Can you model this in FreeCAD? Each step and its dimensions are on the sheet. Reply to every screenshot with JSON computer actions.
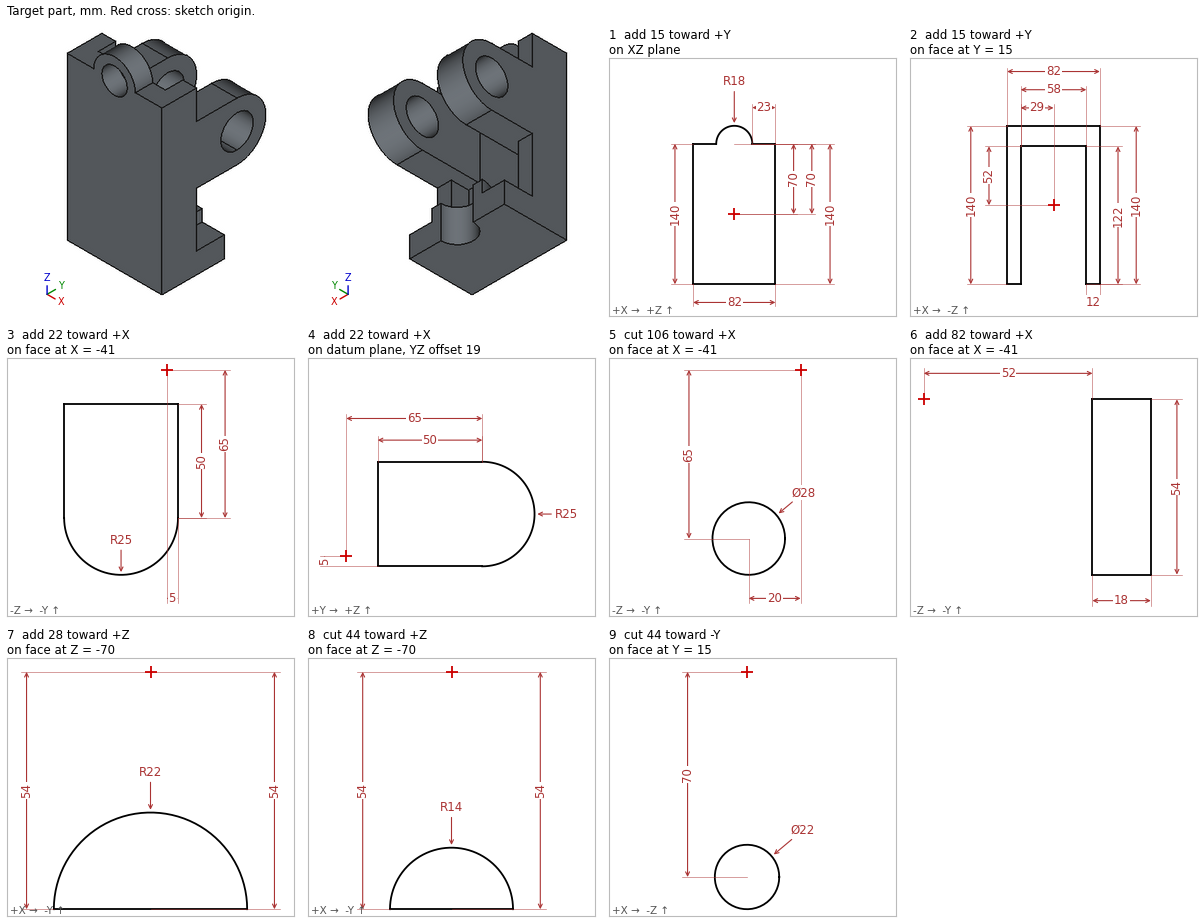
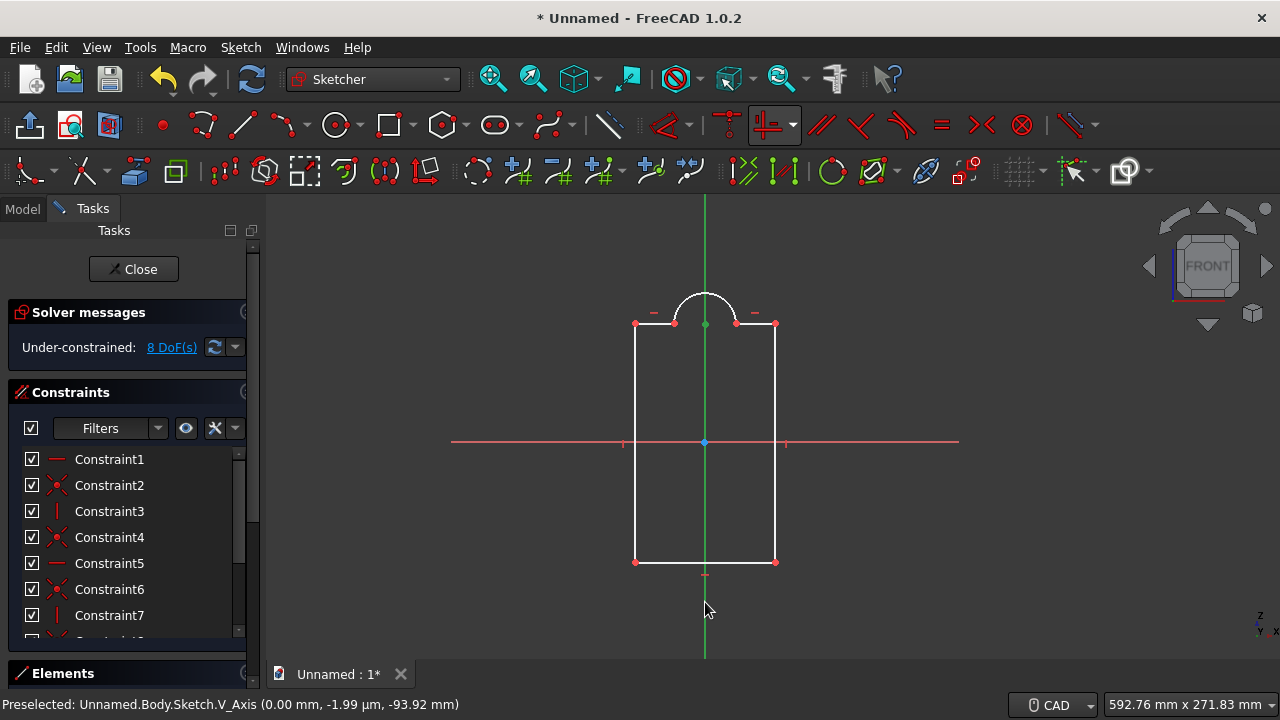
{"action": "left_click", "coordinate": [728, 126]}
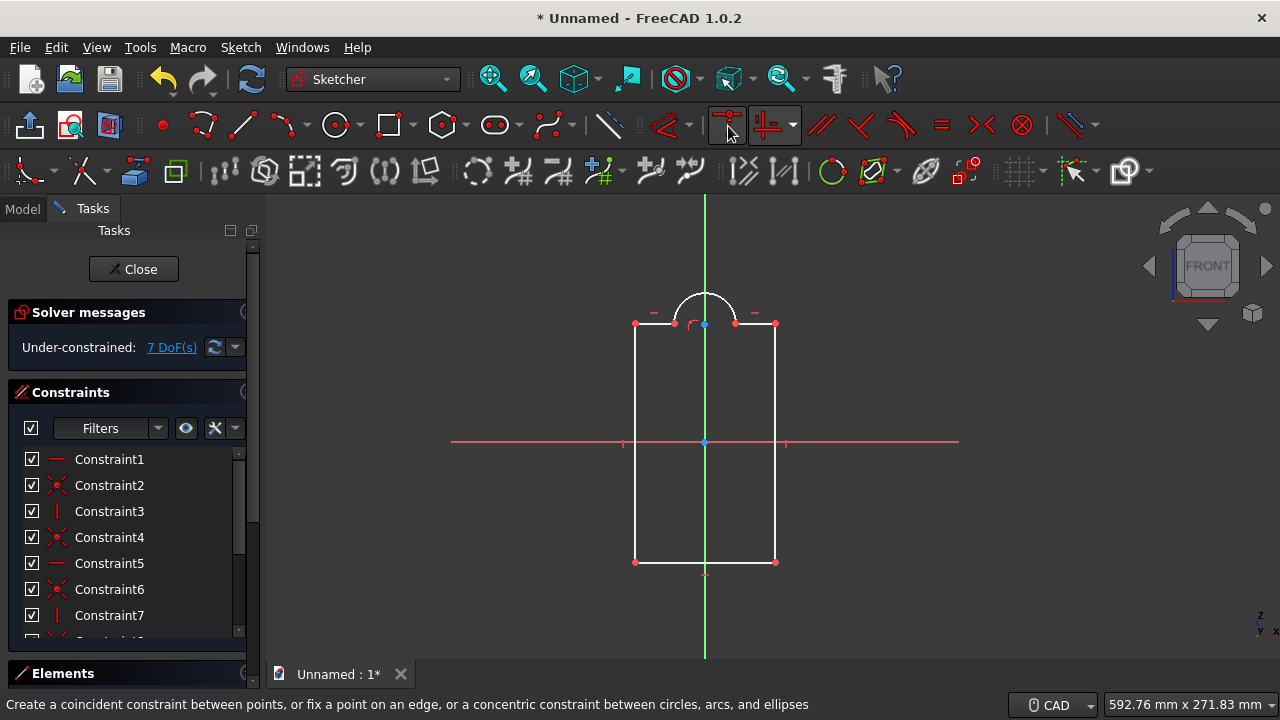
{"action": "scroll", "coordinate": [723, 299], "scroll_direction": "up", "scroll_amount": 2}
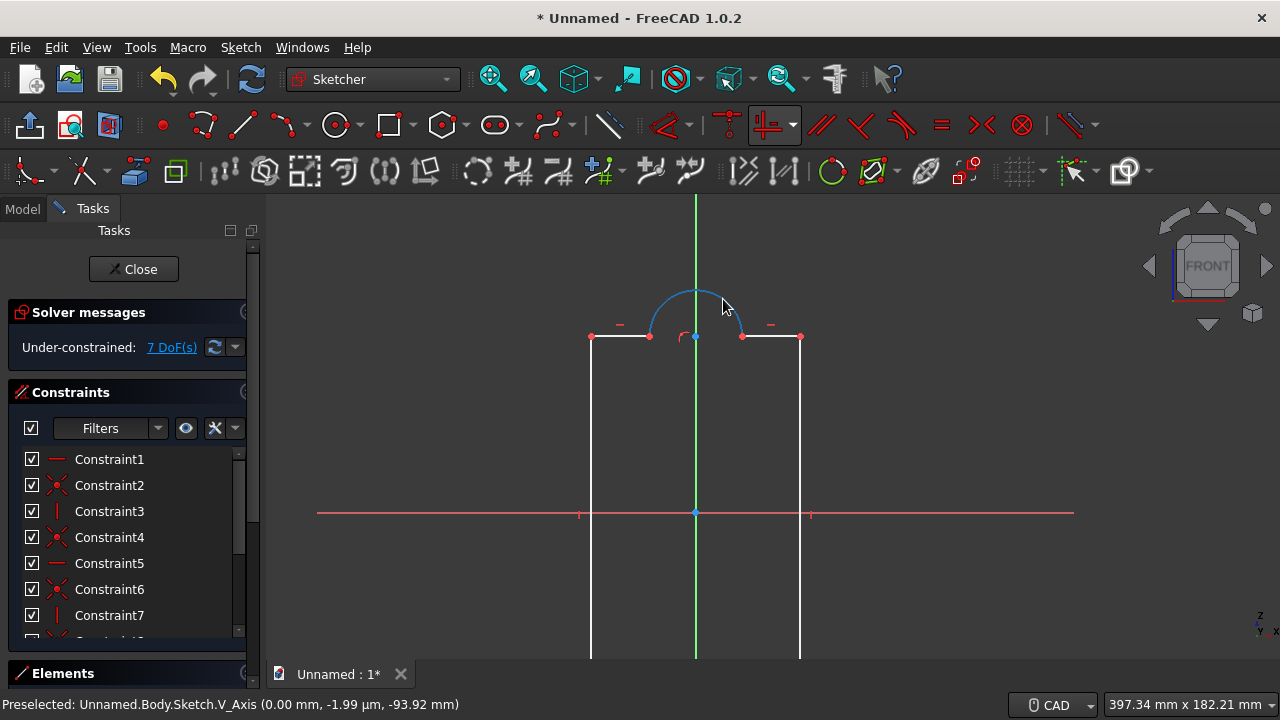
{"action": "left_click", "coordinate": [723, 299]}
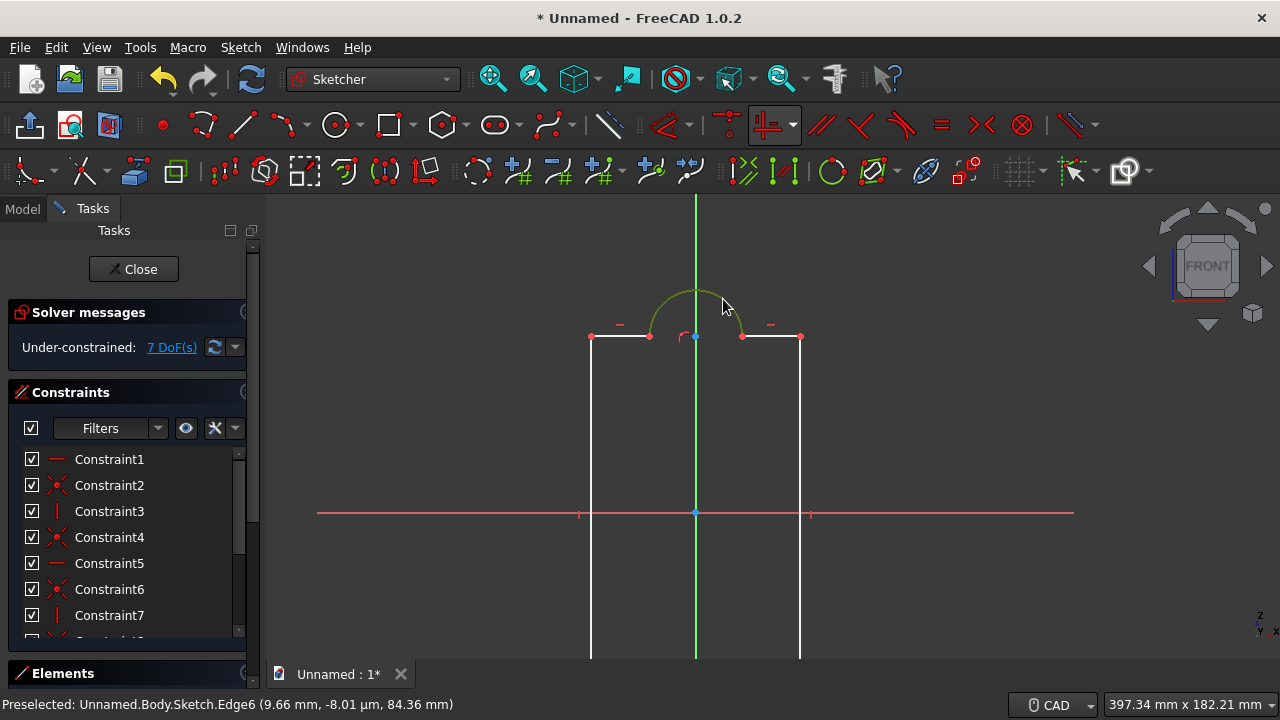
{"action": "key", "text": "k r"}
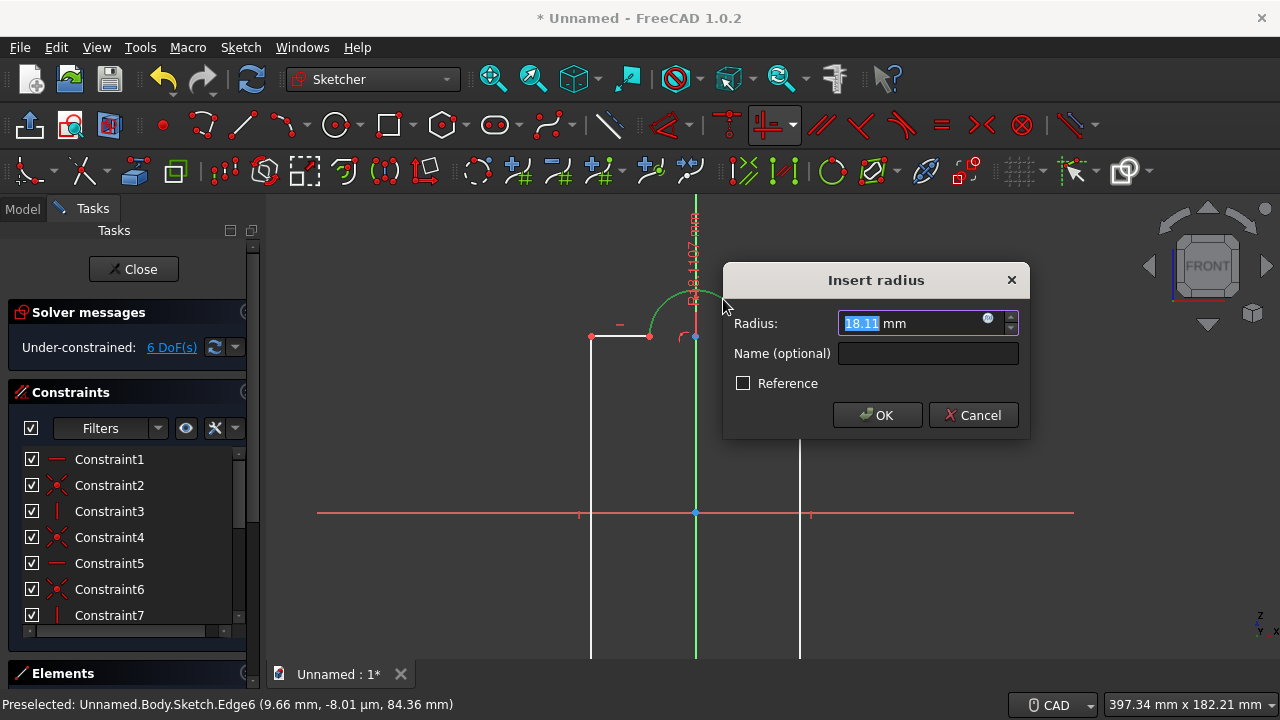
{"action": "type", "text": "18"}
{"action": "key", "text": "Return"}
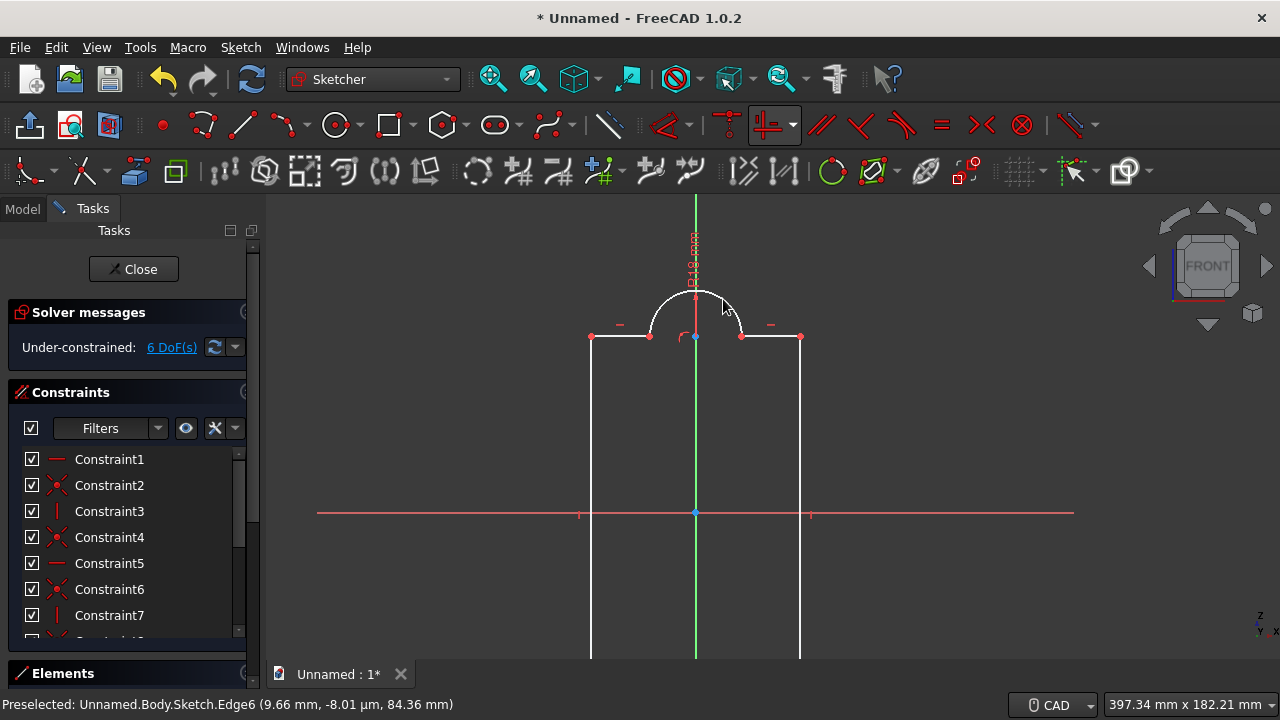
{"action": "left_click", "coordinate": [759, 336]}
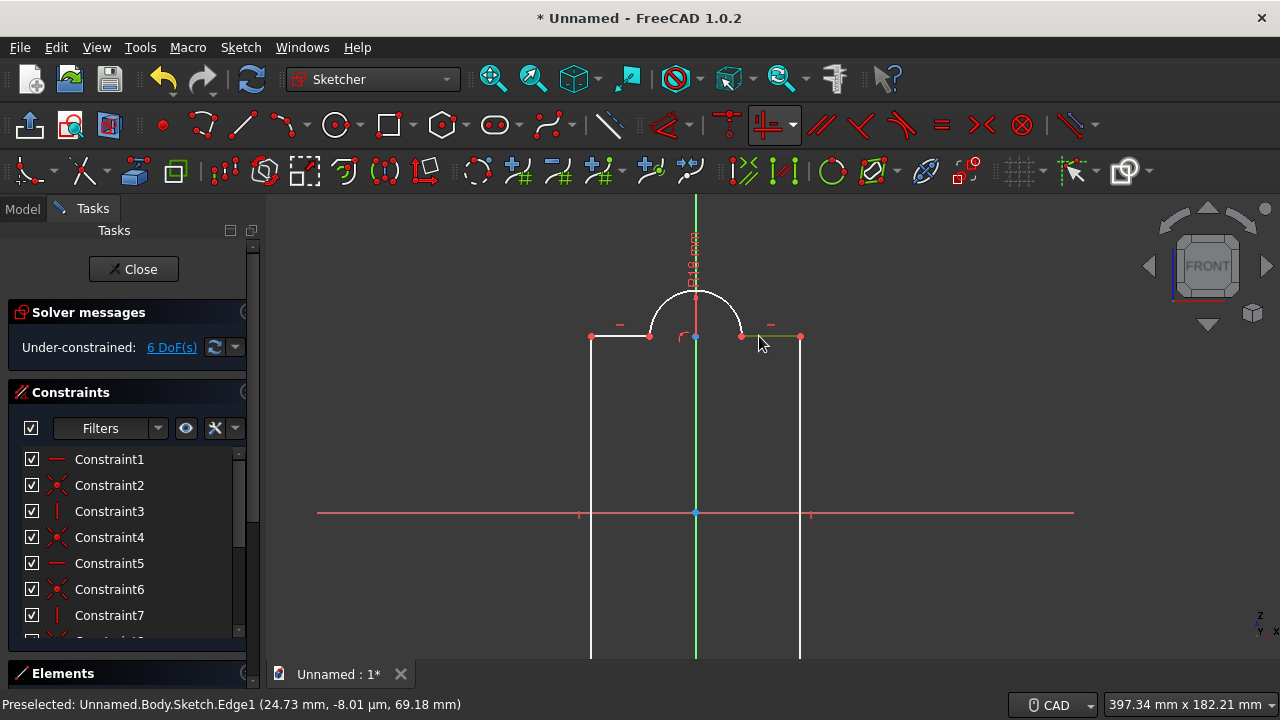
{"action": "key", "text": "l"}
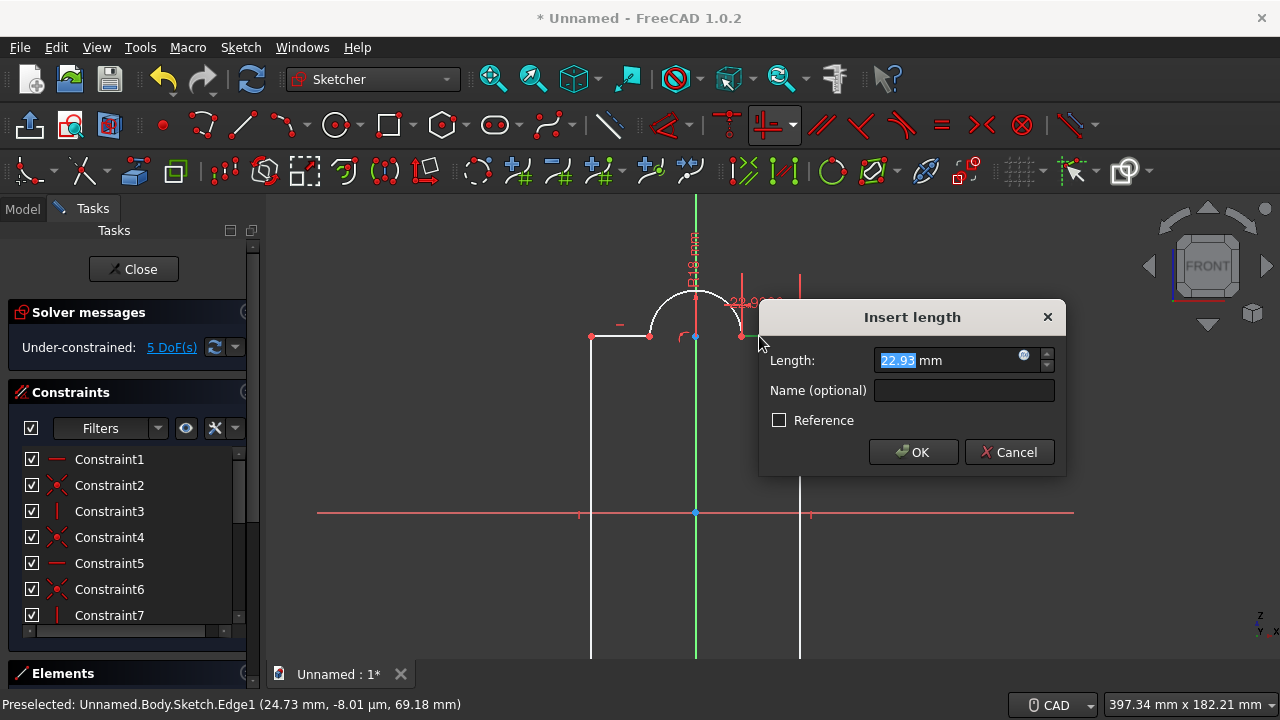
{"action": "type", "text": "23"}
{"action": "key", "text": "Return"}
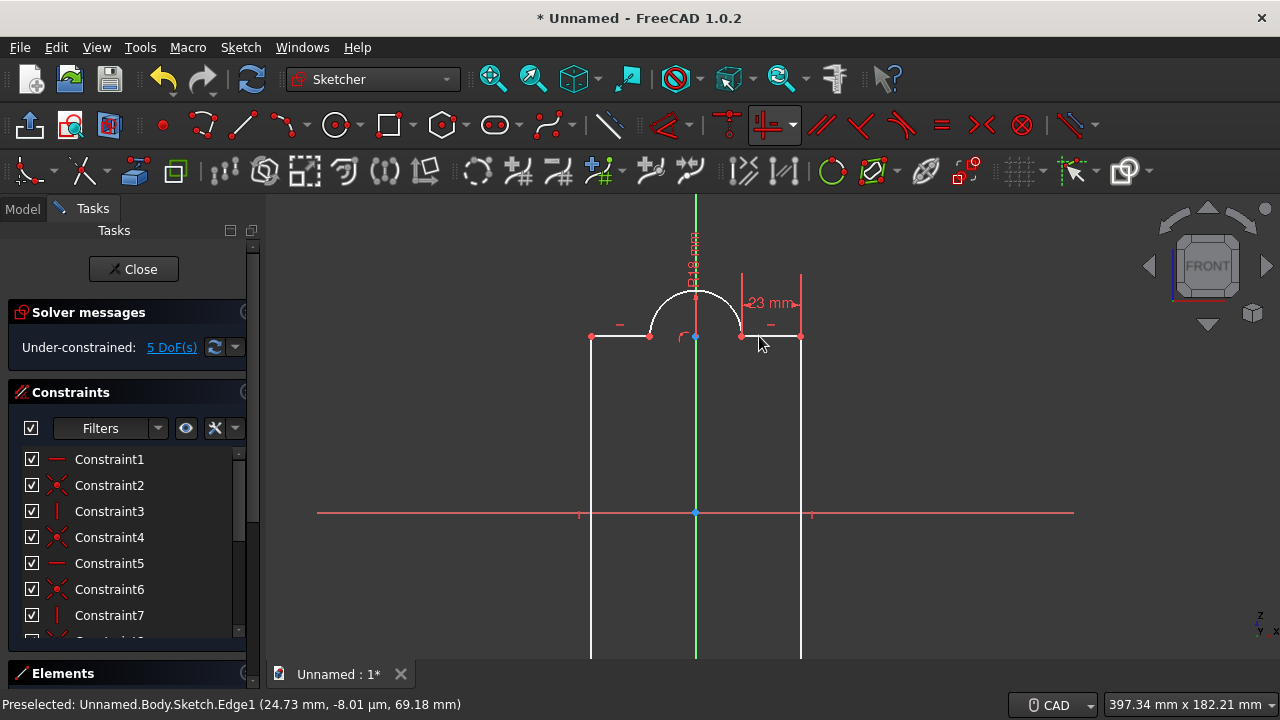
{"action": "scroll", "coordinate": [722, 298], "scroll_direction": "down", "scroll_amount": 2}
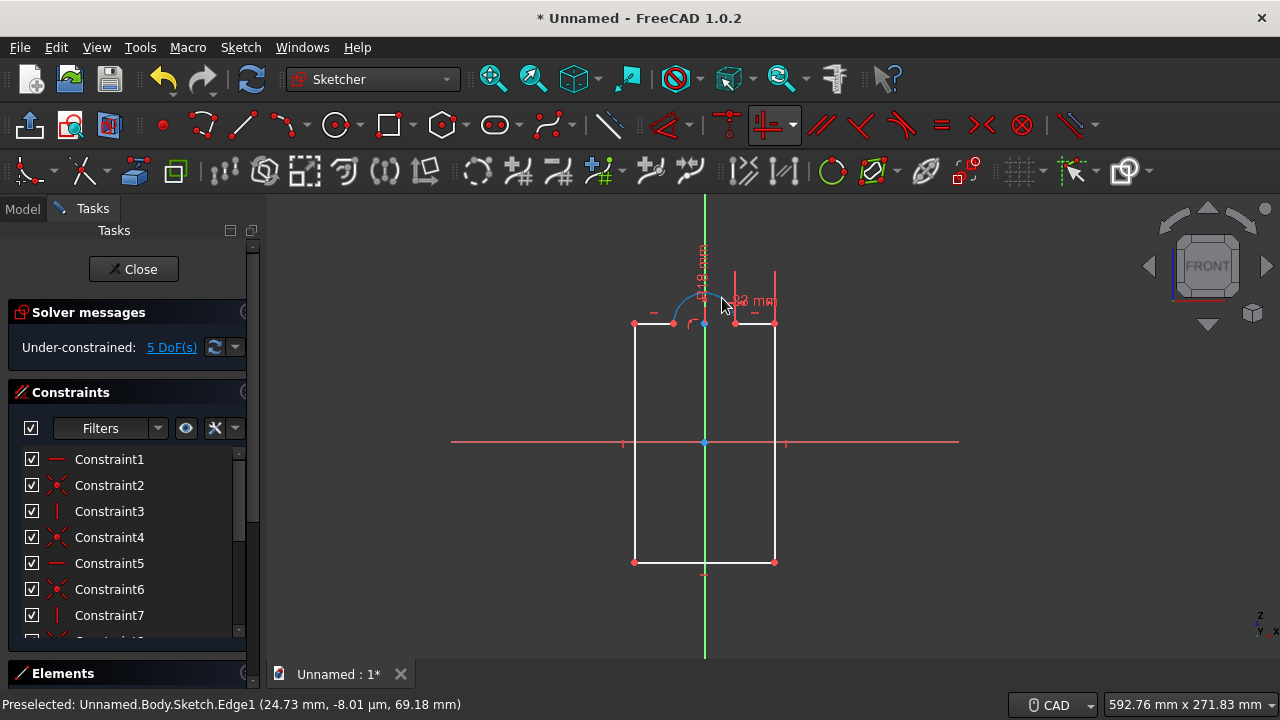
{"action": "left_click", "coordinate": [733, 563]}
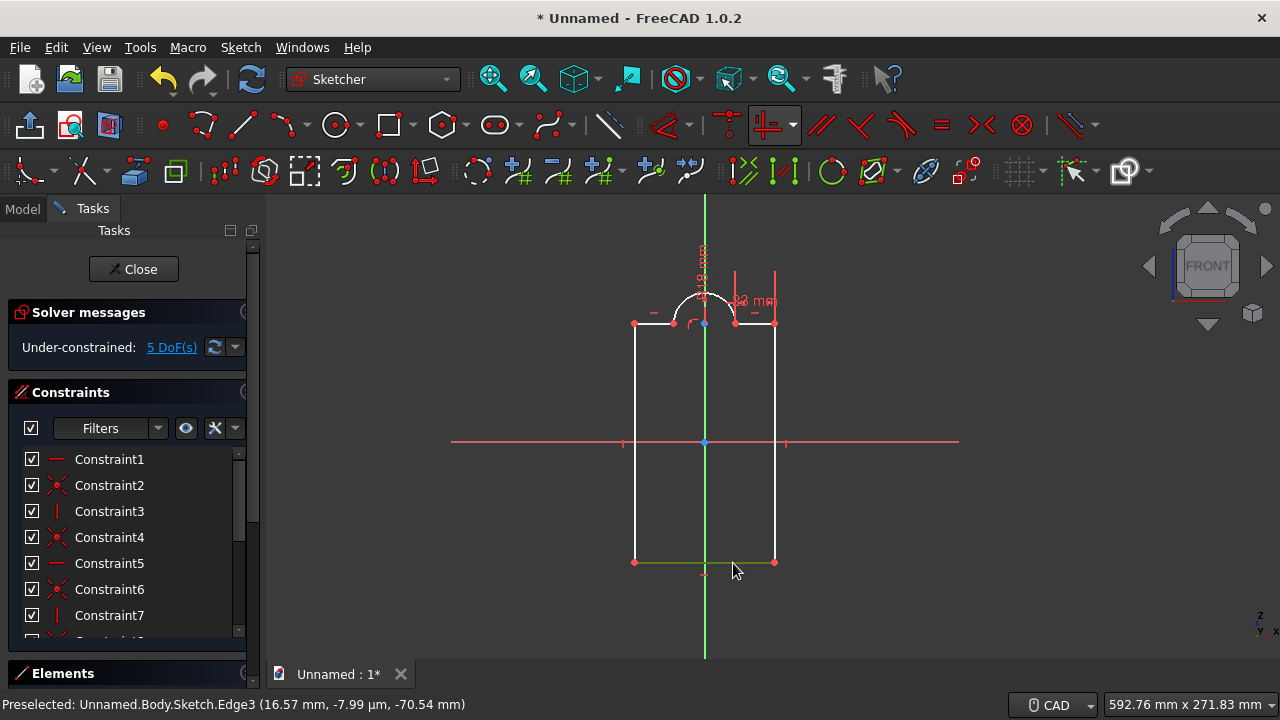
{"action": "key", "text": "l"}